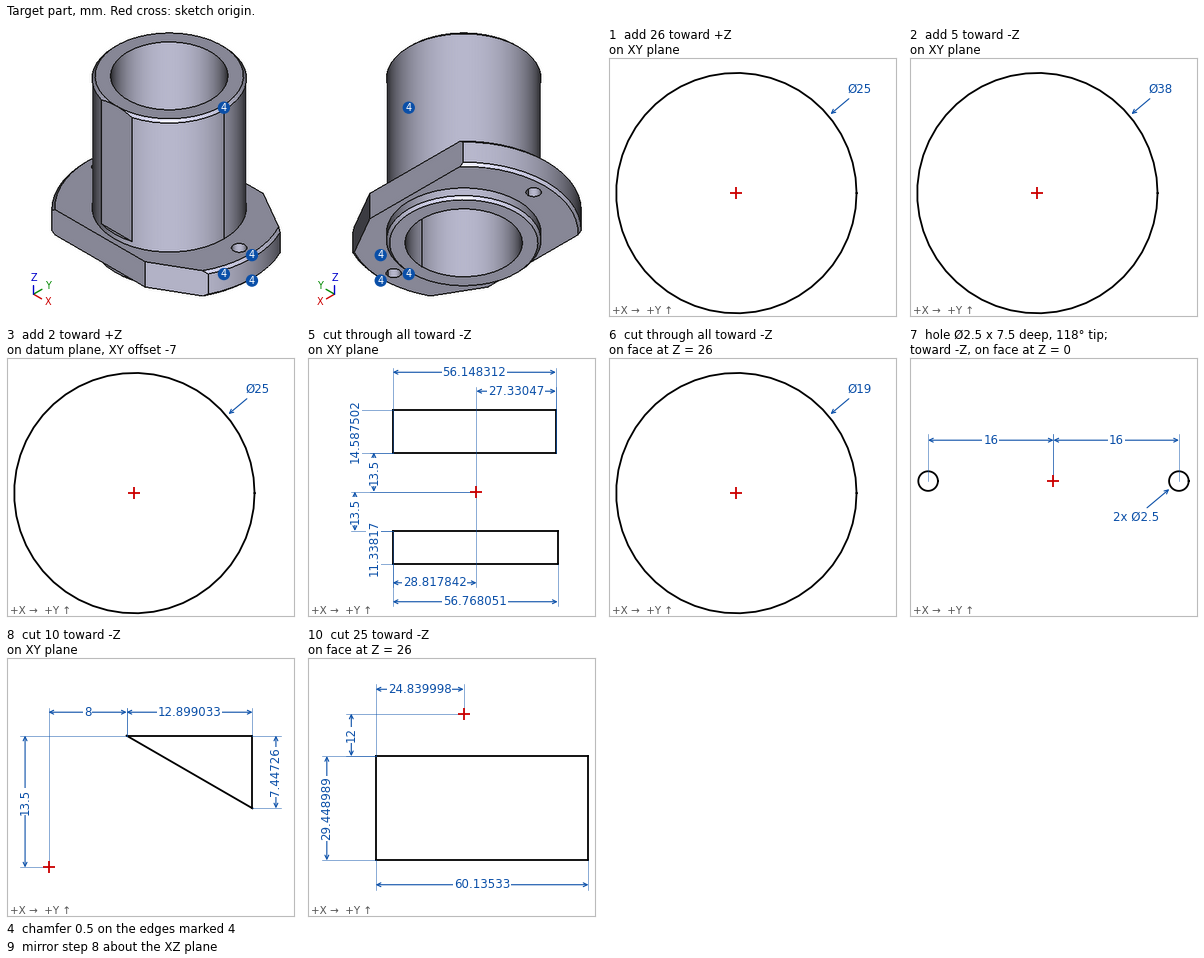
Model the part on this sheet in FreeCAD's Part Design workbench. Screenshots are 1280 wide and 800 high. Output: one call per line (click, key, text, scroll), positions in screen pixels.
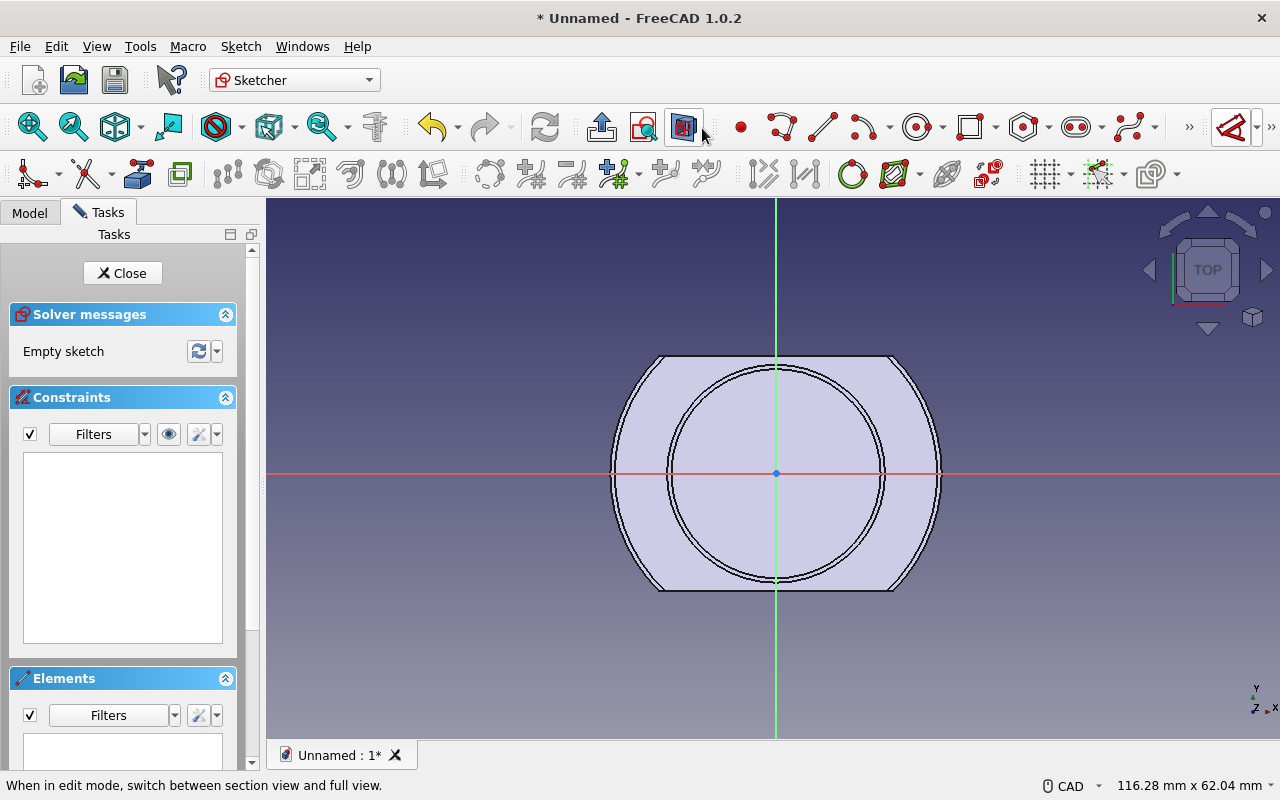
scroll(834, 478, up, 4)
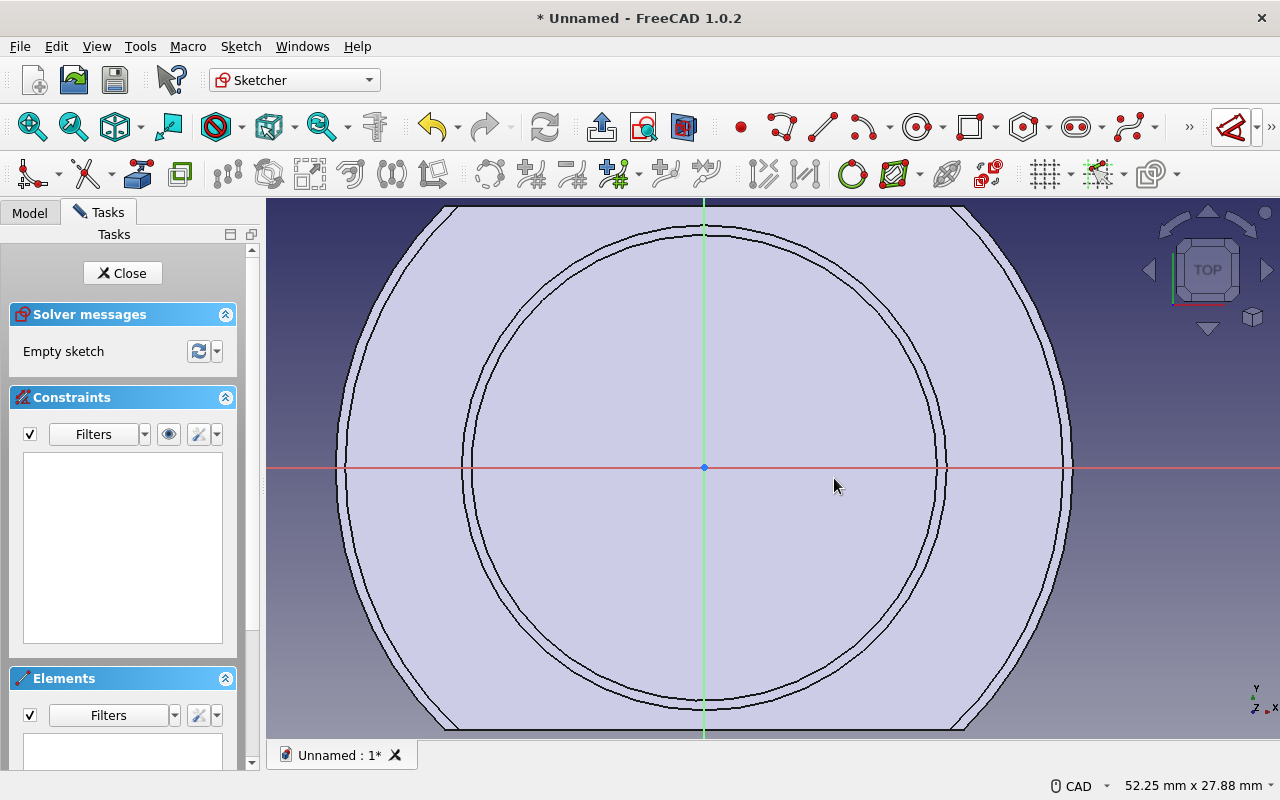
key(g)
key(c)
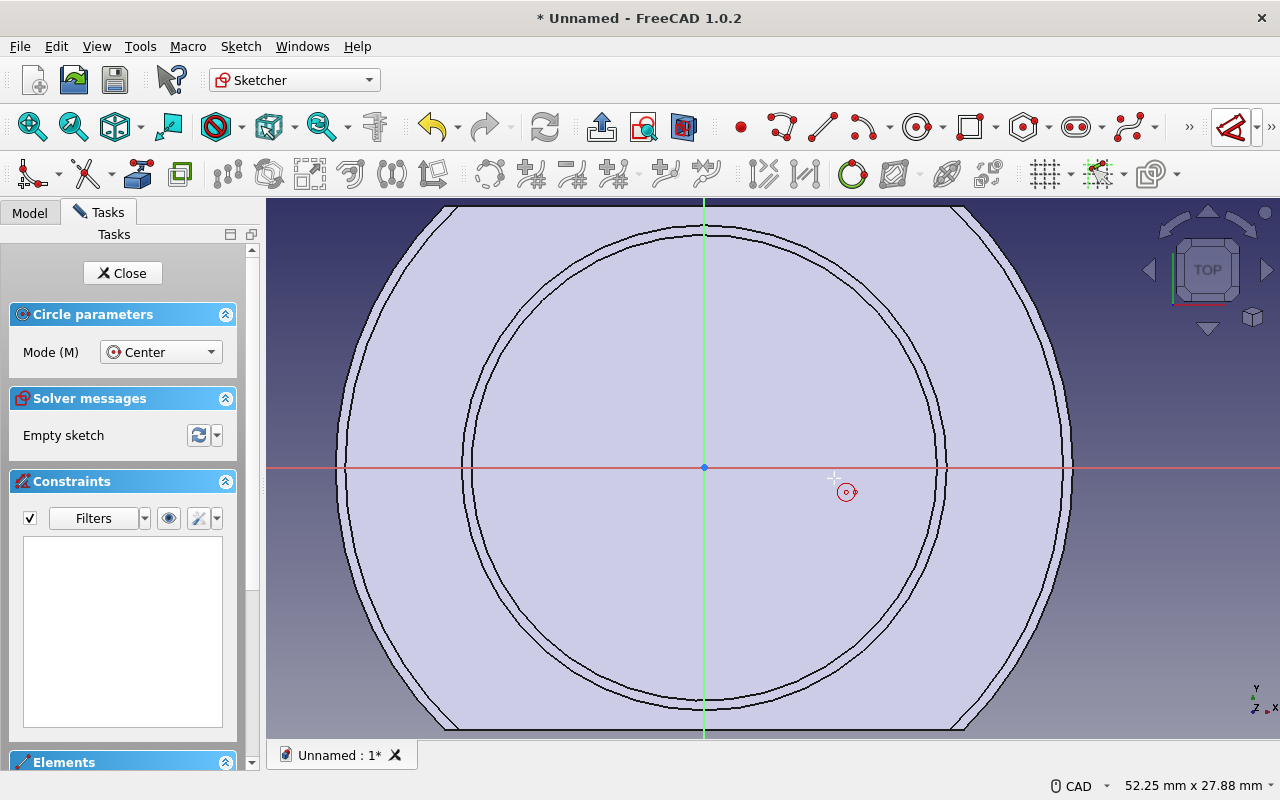
click(704, 468)
click(835, 337)
key(Escape)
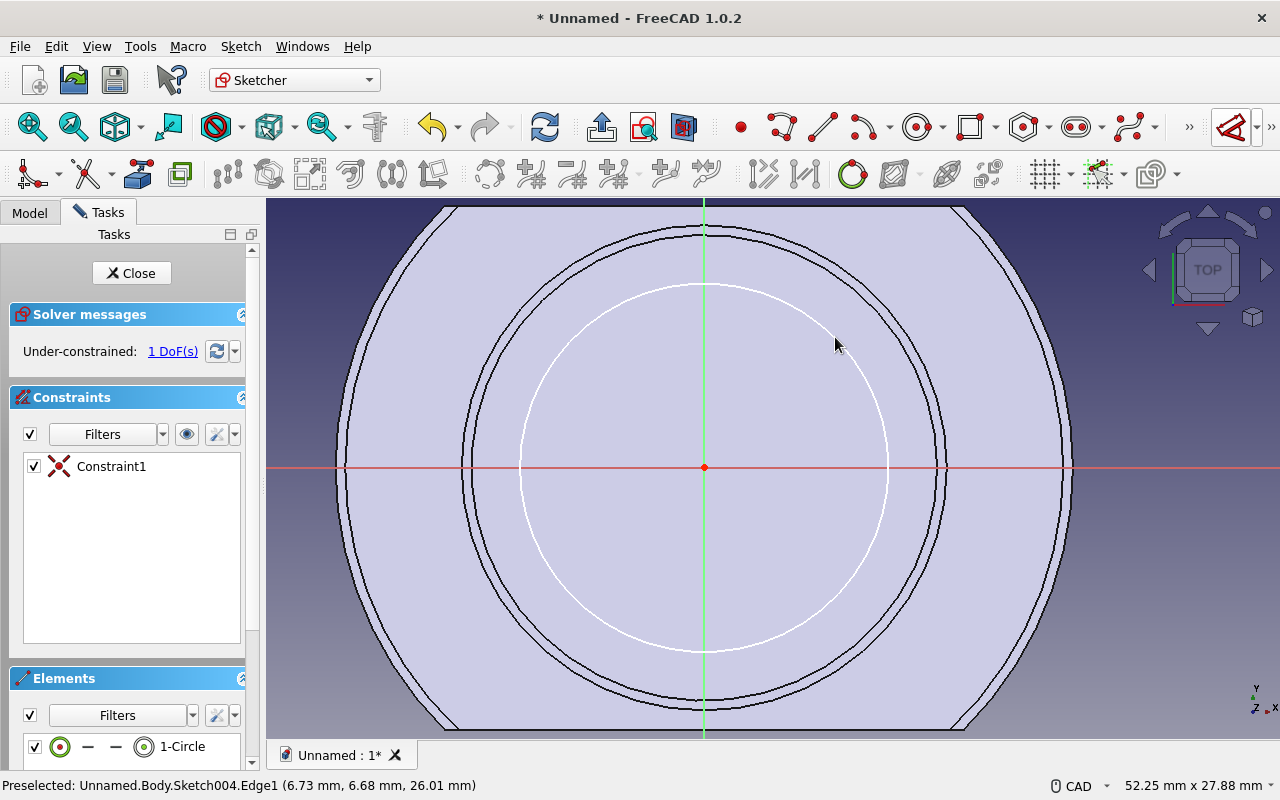
click(834, 337)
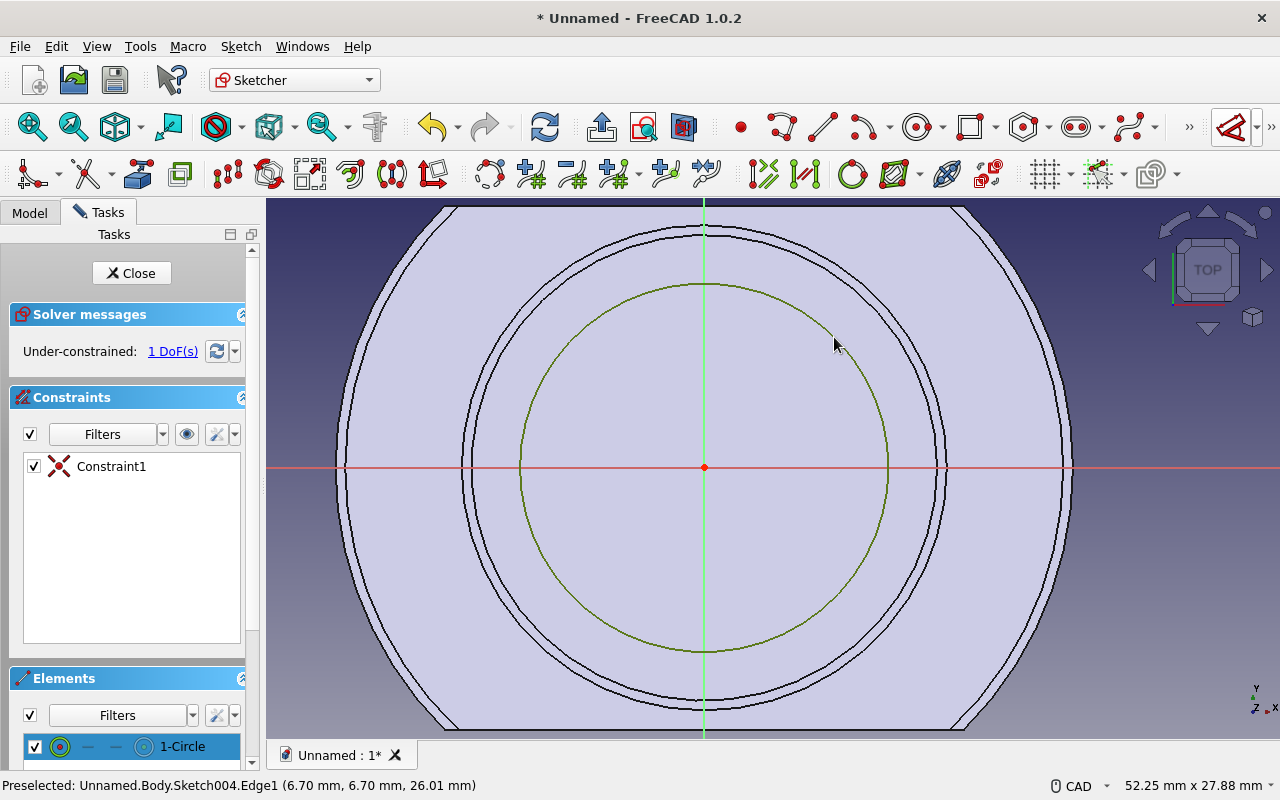
click(1256, 128)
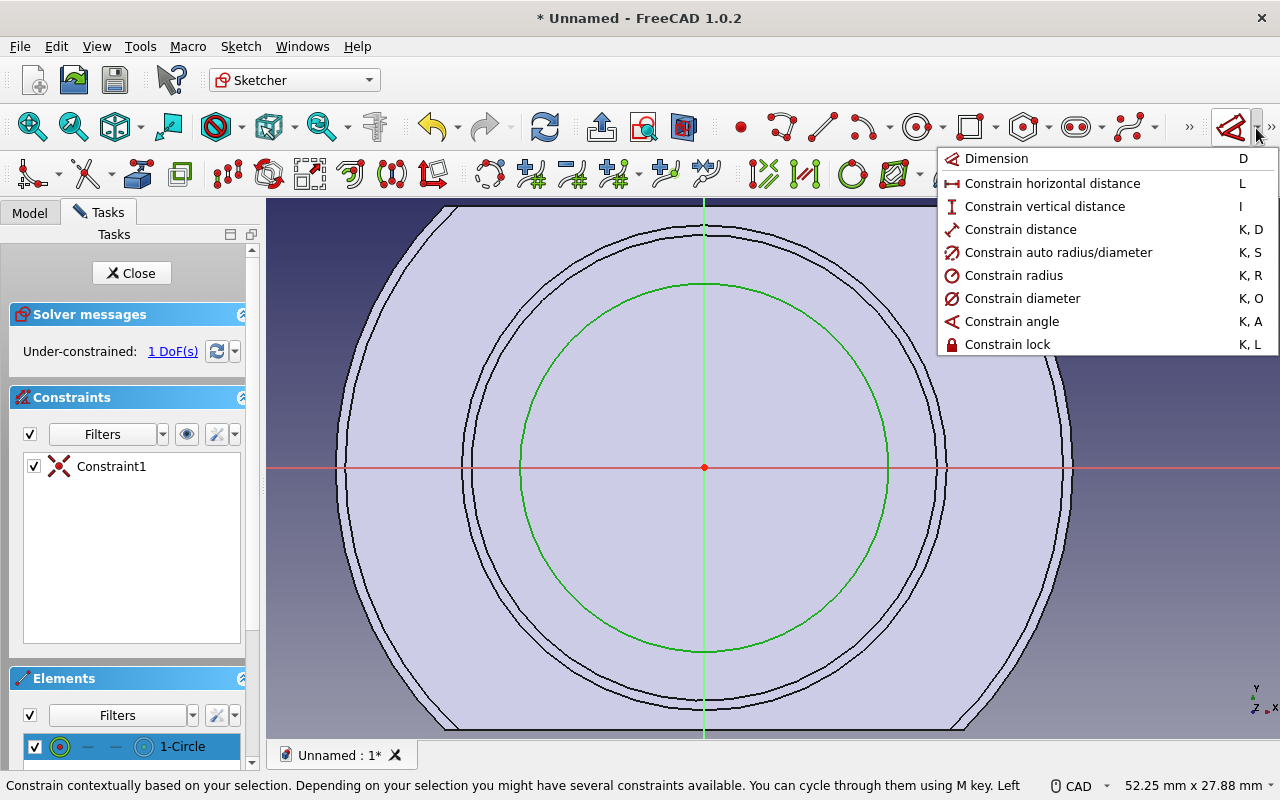
click(1108, 298)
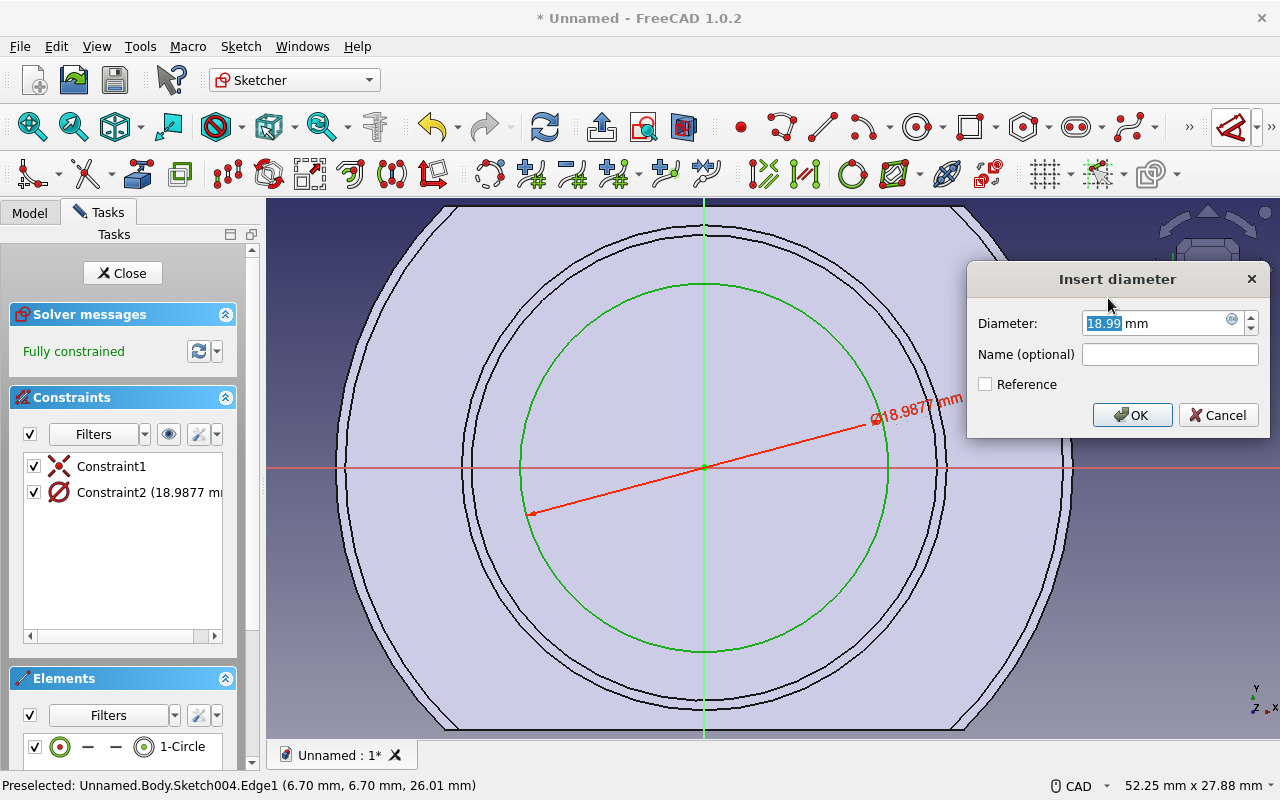
text(19)
key(Return)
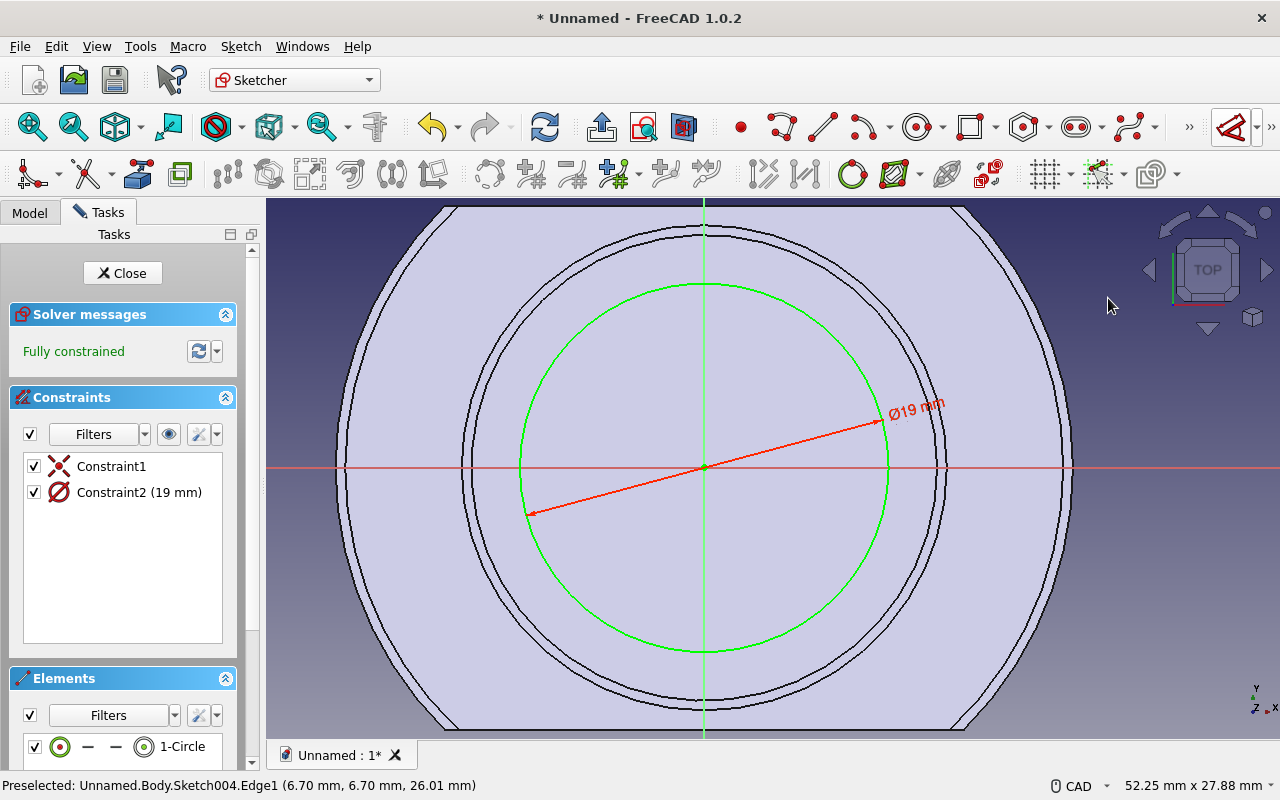
click(123, 273)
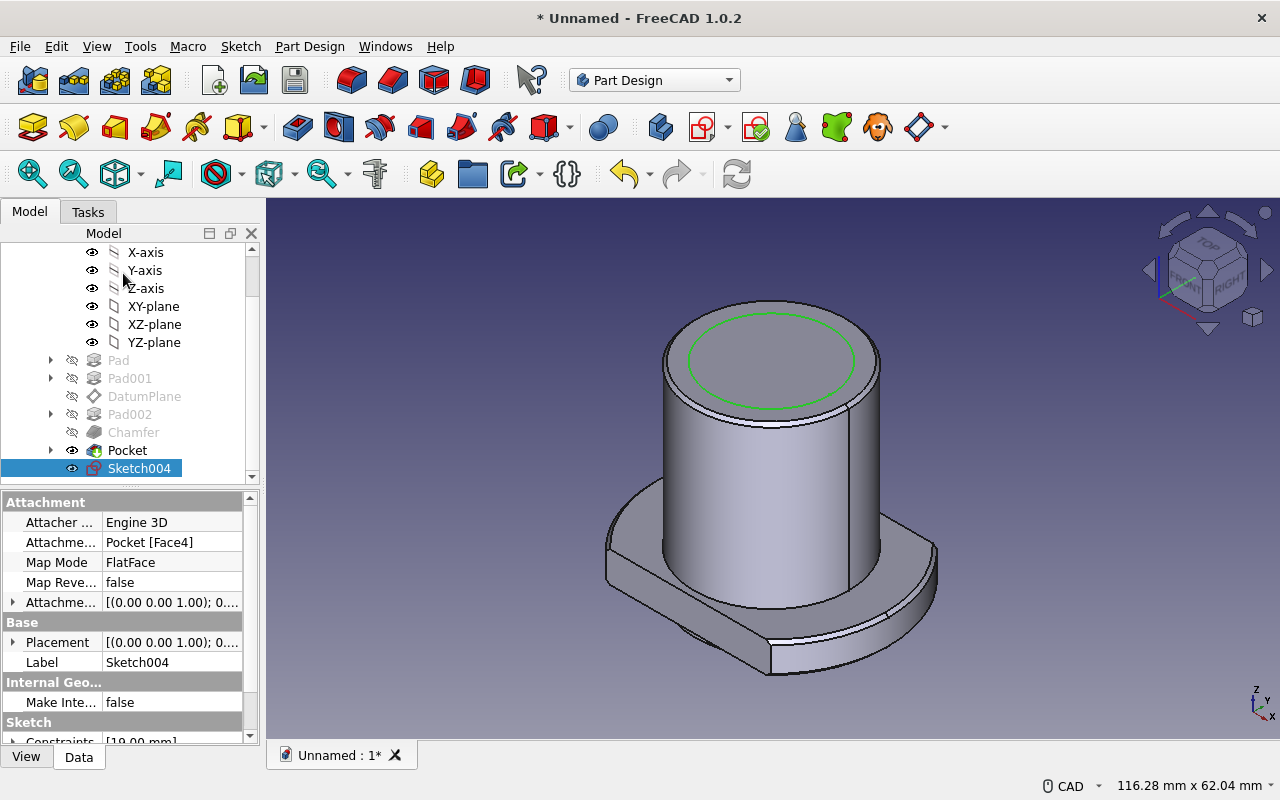
click(298, 128)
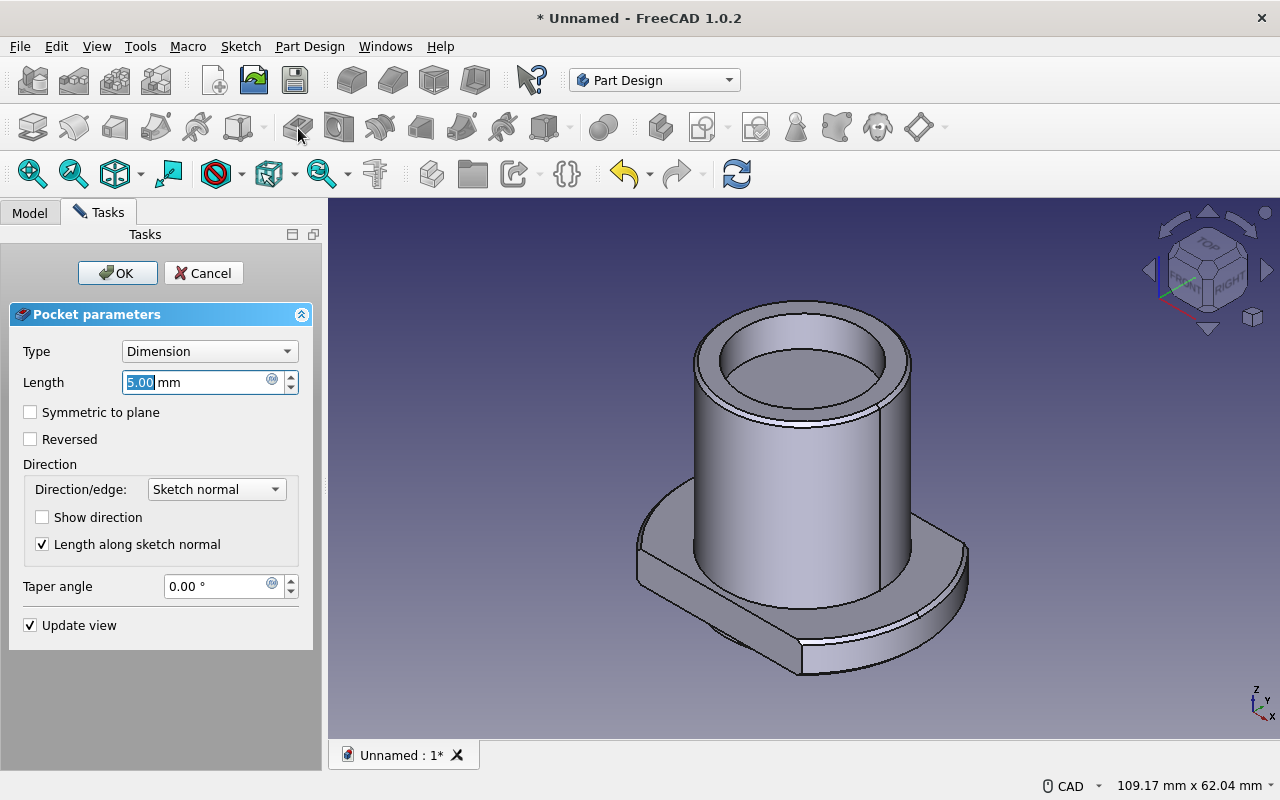
click(210, 352)